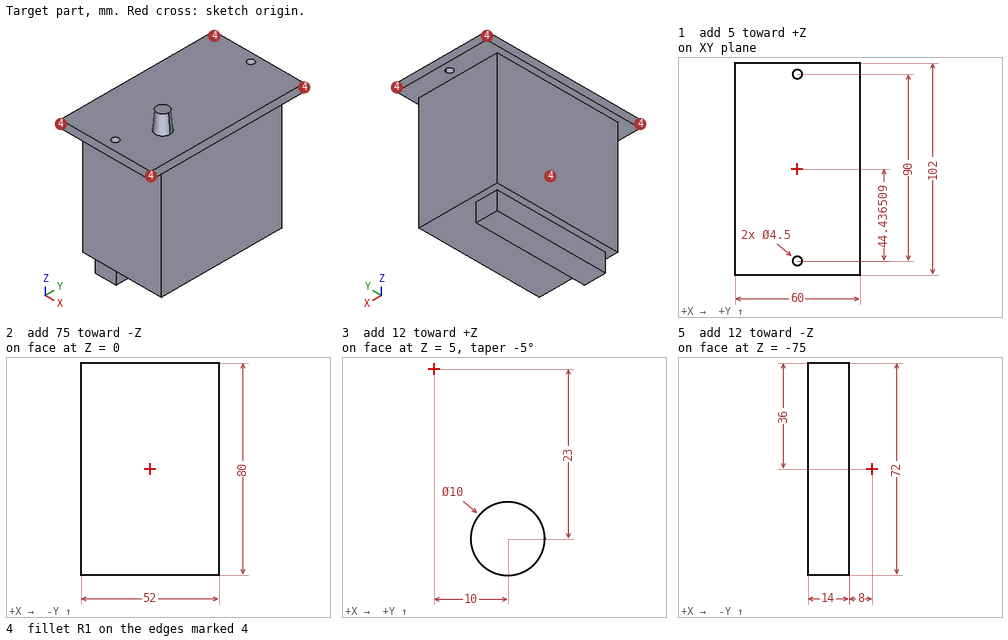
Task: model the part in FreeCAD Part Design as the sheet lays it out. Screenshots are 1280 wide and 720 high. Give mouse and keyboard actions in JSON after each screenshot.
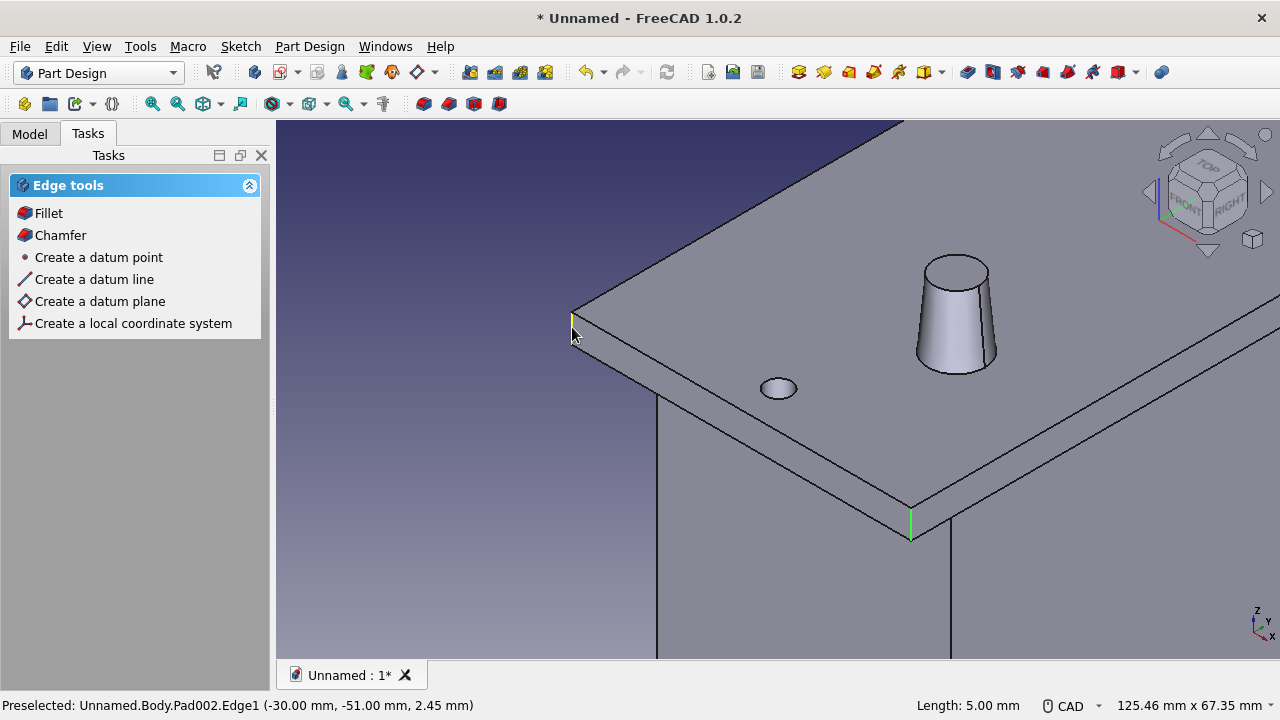
{"action": "left_click", "coordinate": [153, 104]}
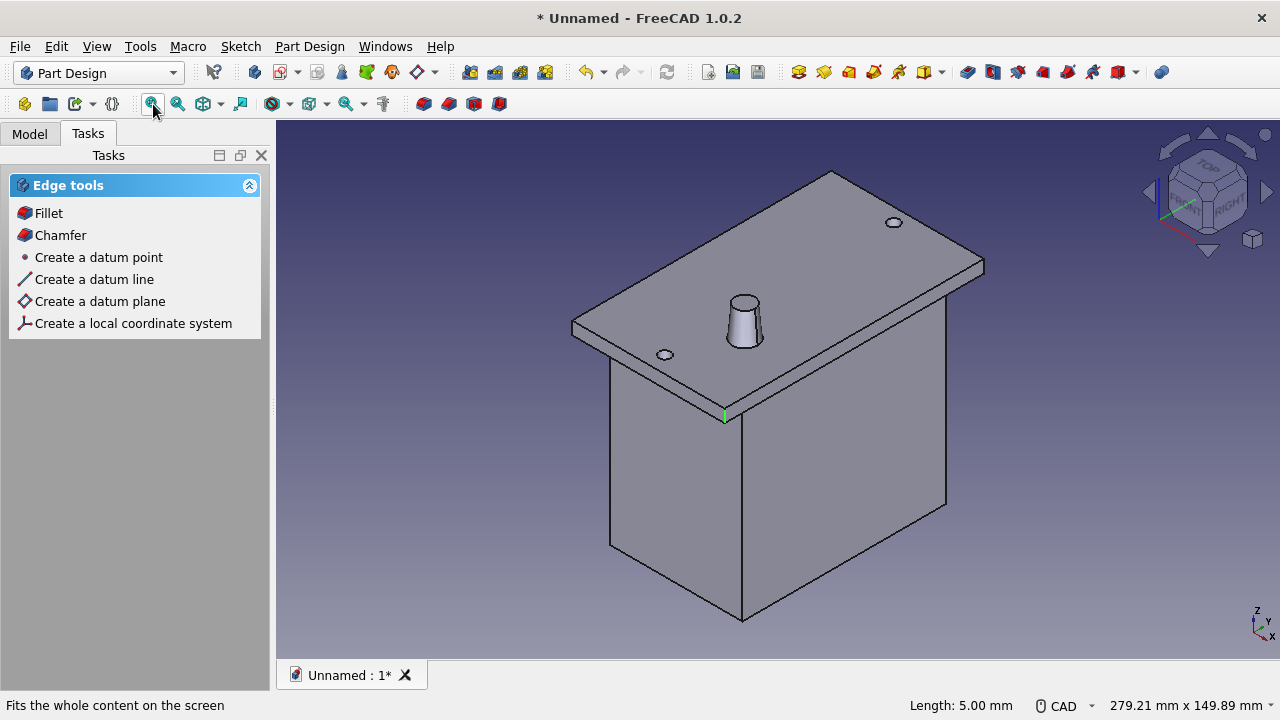
{"action": "key", "text": "1"}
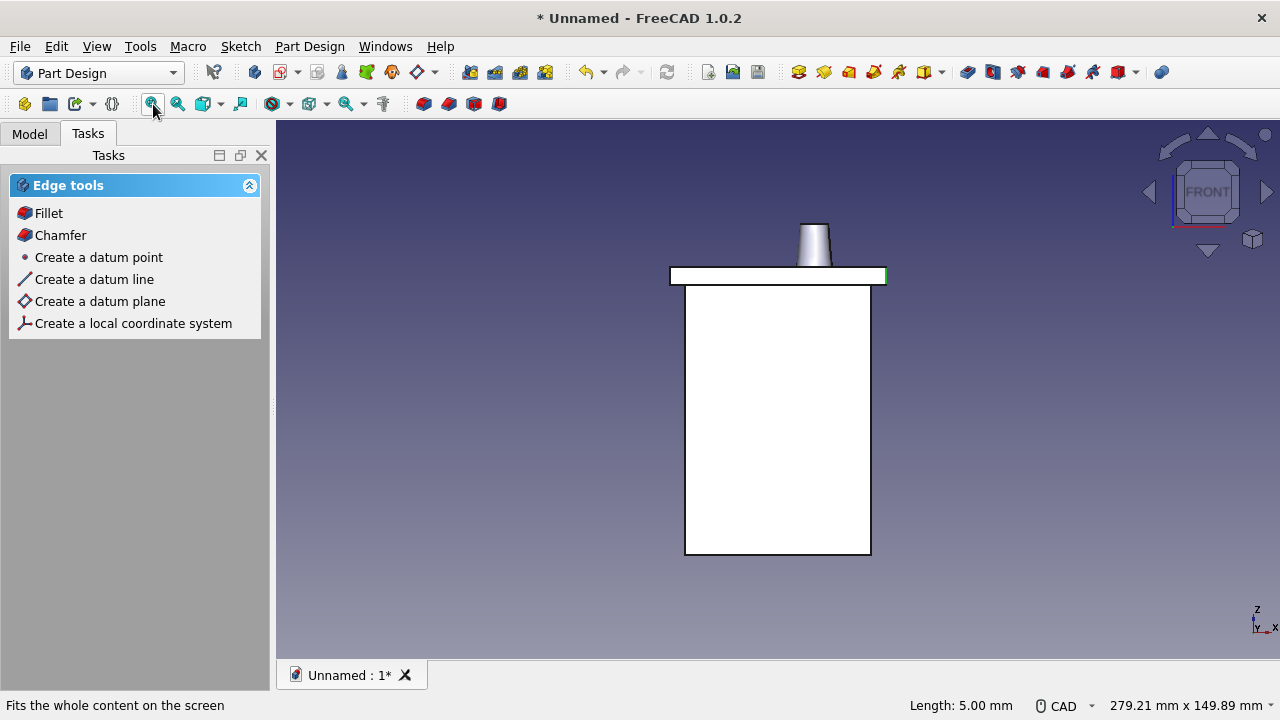
{"action": "left_click", "coordinate": [670, 275], "text": "ctrl"}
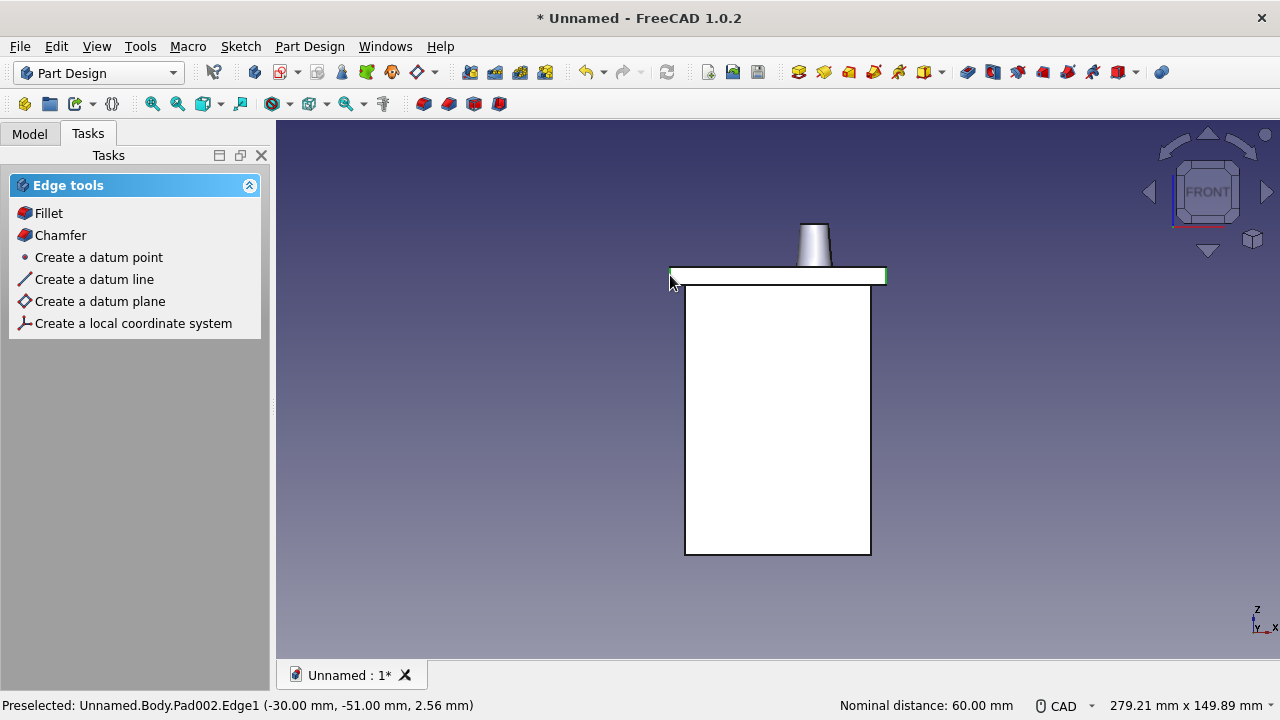
{"action": "scroll", "coordinate": [670, 275], "scroll_direction": "up", "scroll_amount": 4}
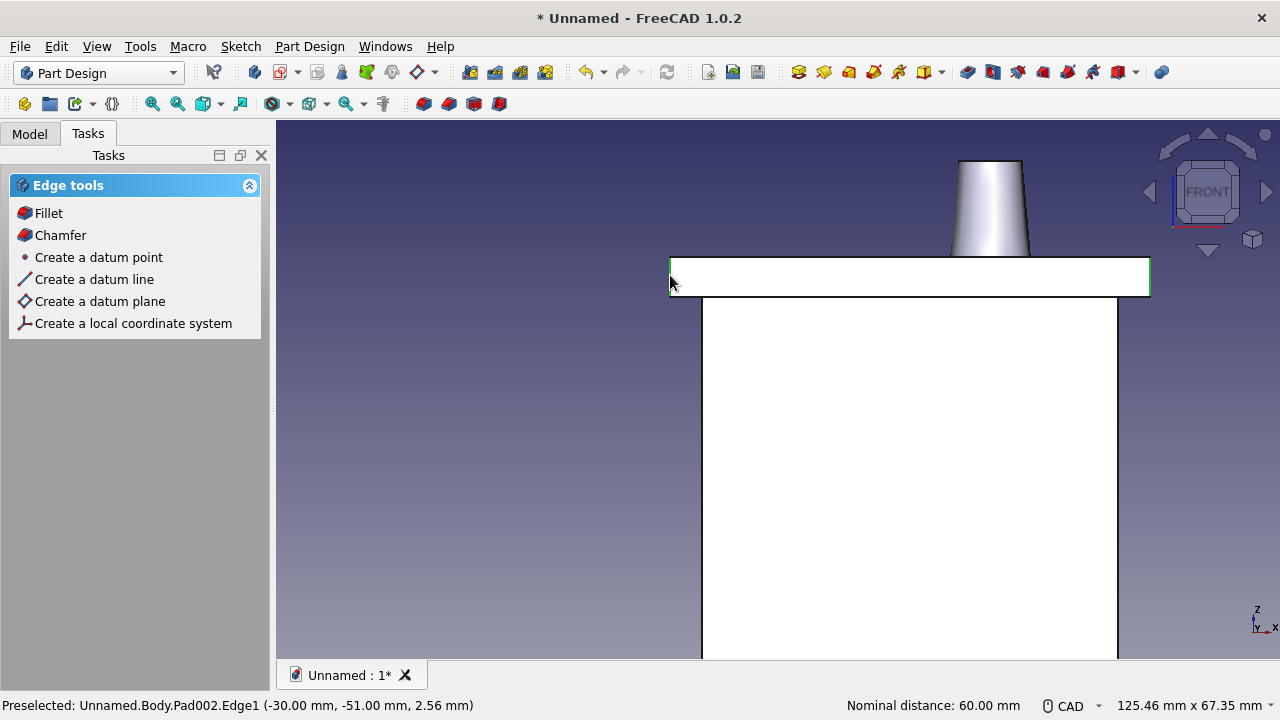
{"action": "key", "text": "v f"}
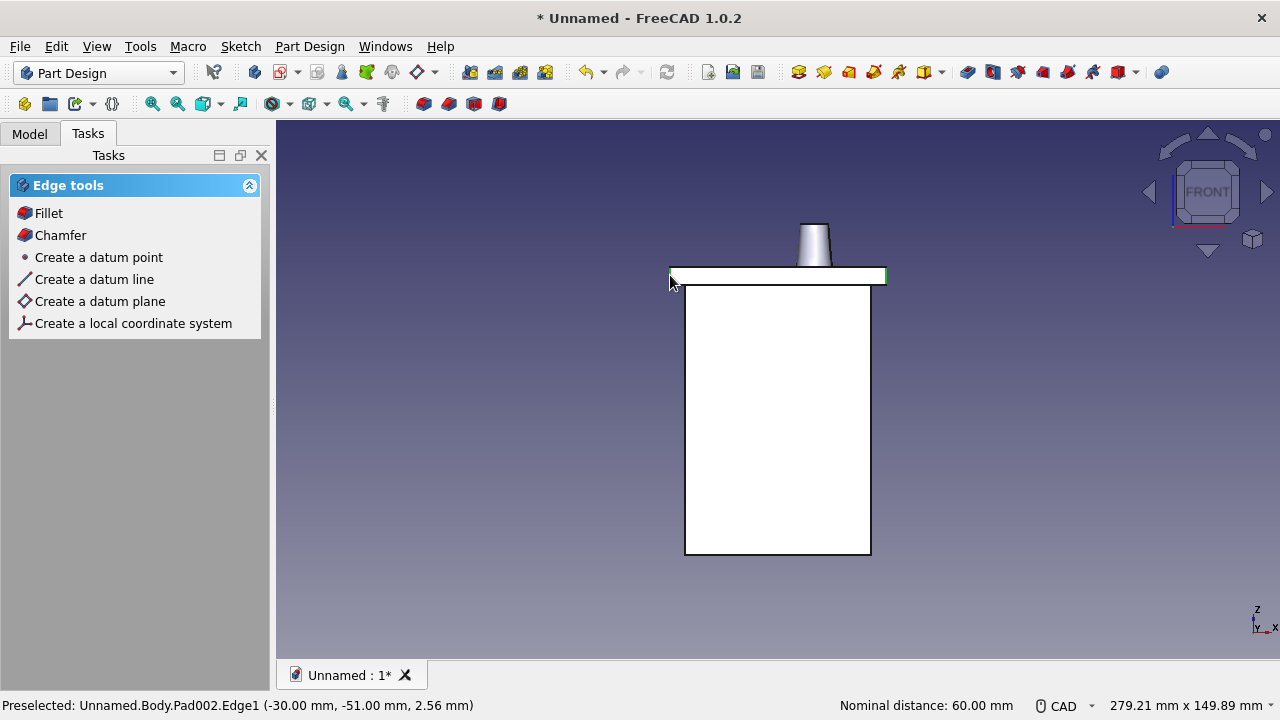
{"action": "key", "text": "3"}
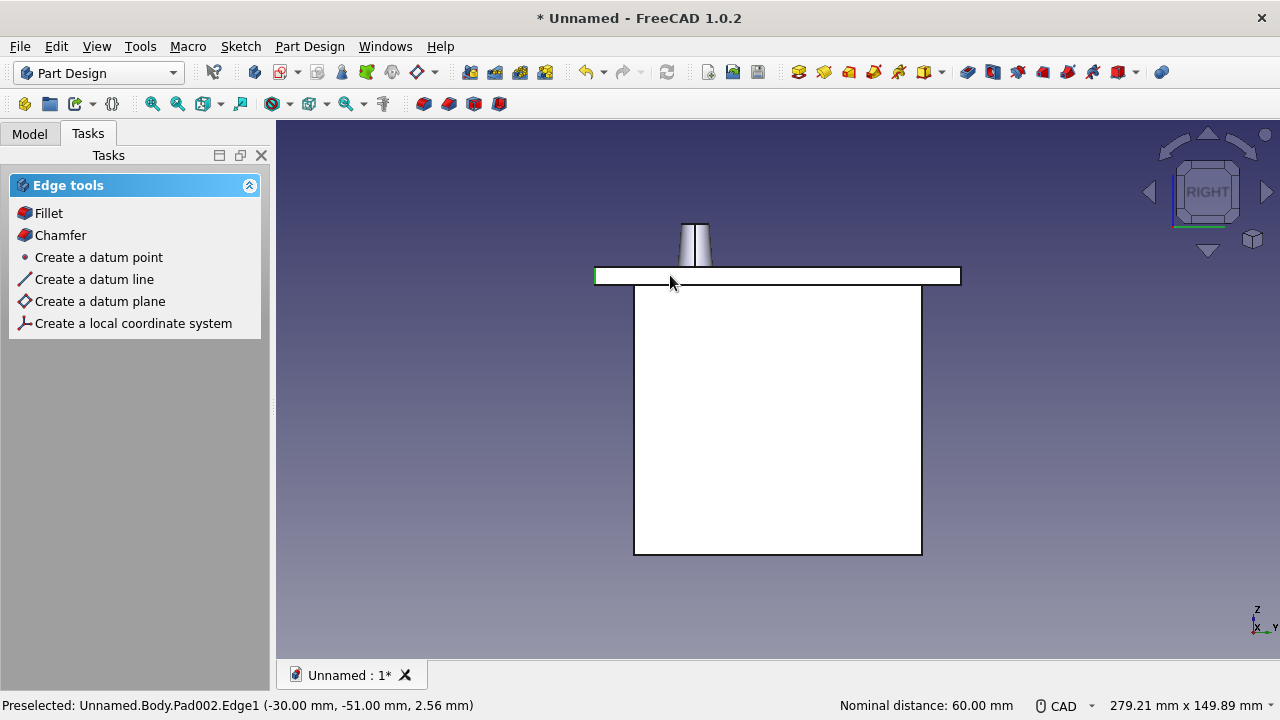
{"action": "left_click", "coordinate": [961, 275], "text": "ctrl"}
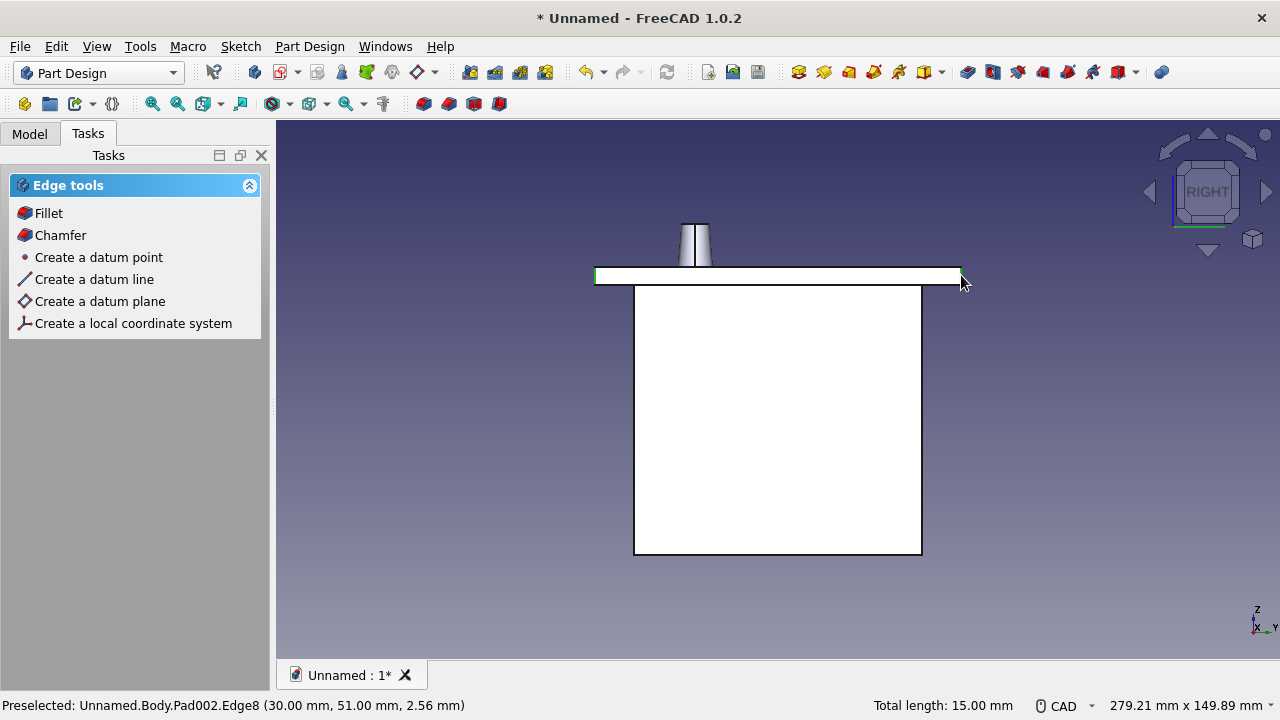
{"action": "scroll", "coordinate": [961, 275], "scroll_direction": "up", "scroll_amount": 4}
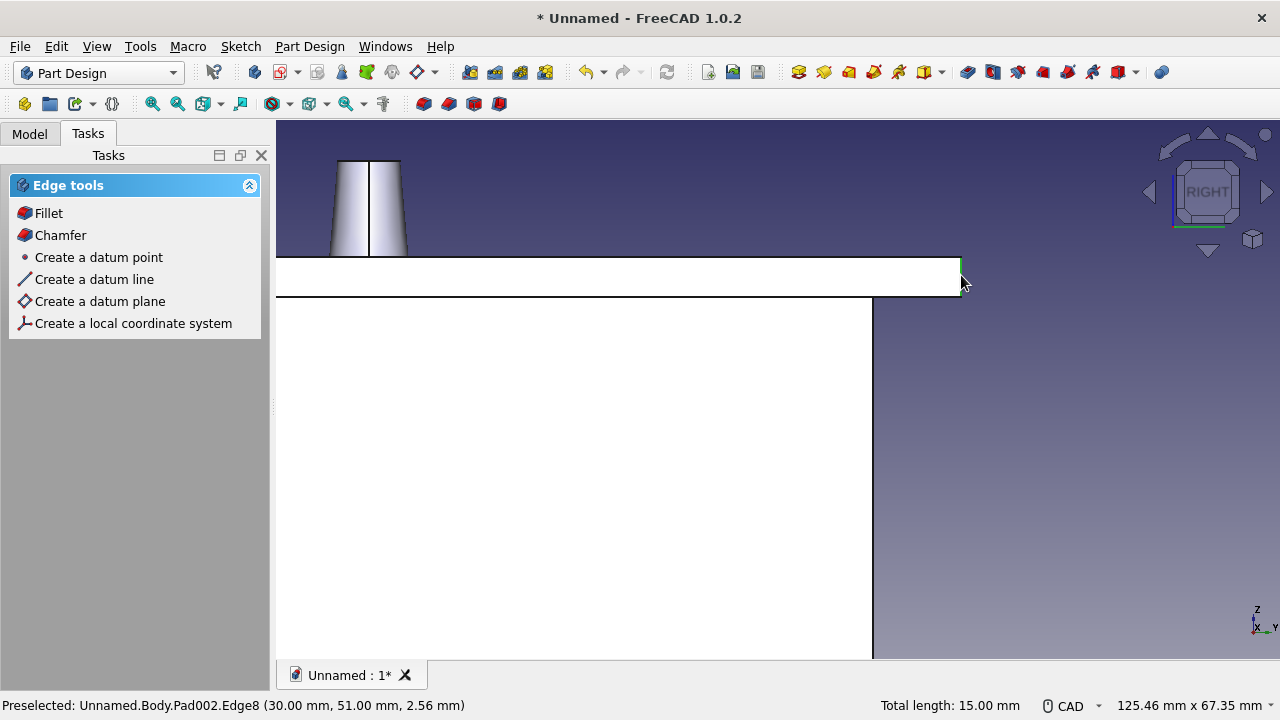
{"action": "left_click", "coordinate": [153, 104]}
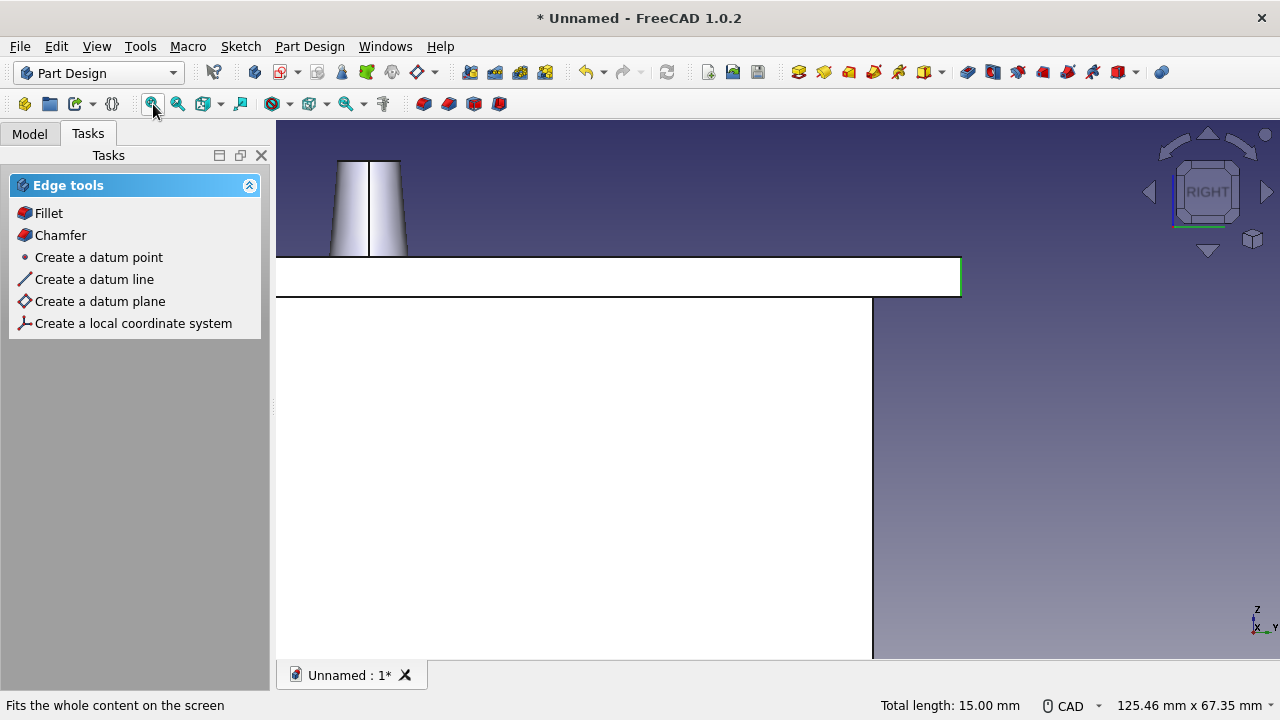
{"action": "key", "text": "5"}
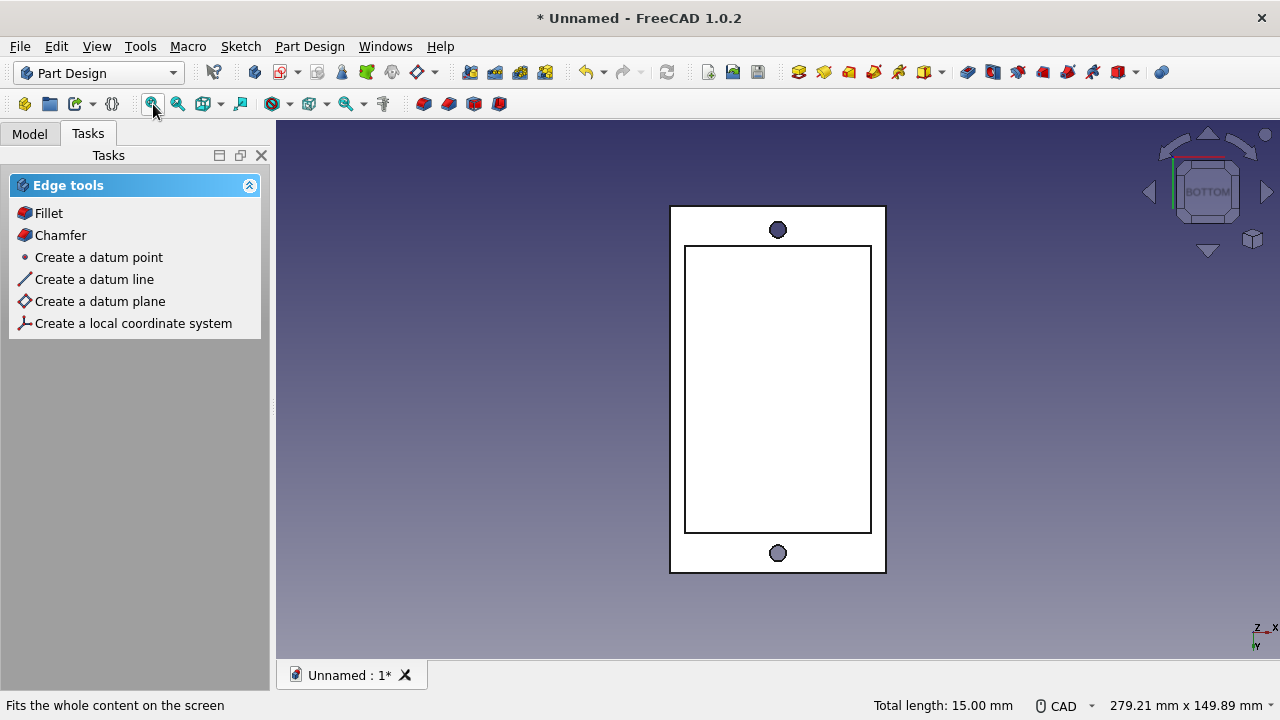
{"action": "scroll", "coordinate": [670, 572], "scroll_direction": "up", "scroll_amount": 4}